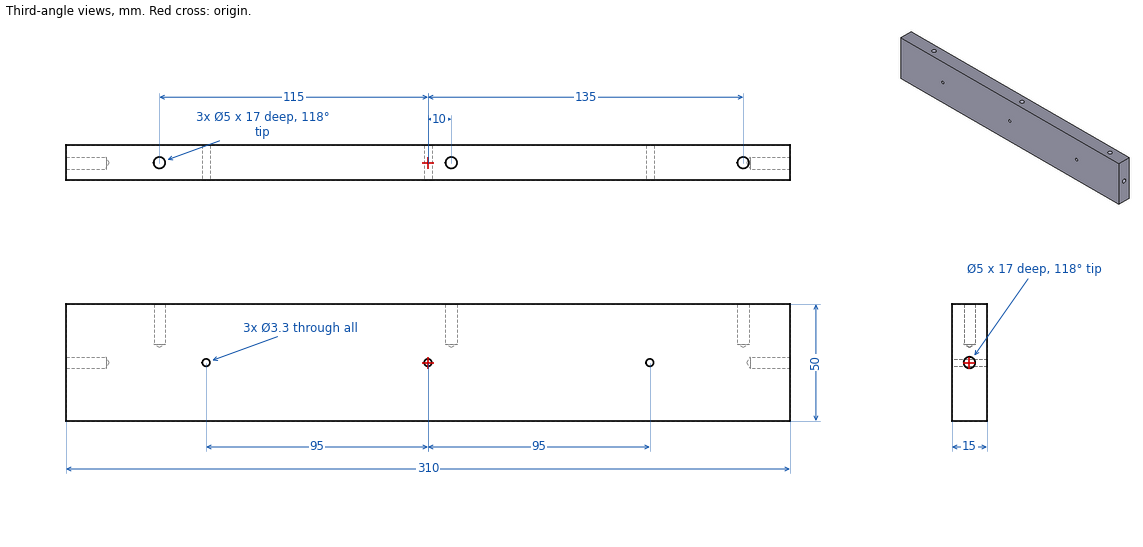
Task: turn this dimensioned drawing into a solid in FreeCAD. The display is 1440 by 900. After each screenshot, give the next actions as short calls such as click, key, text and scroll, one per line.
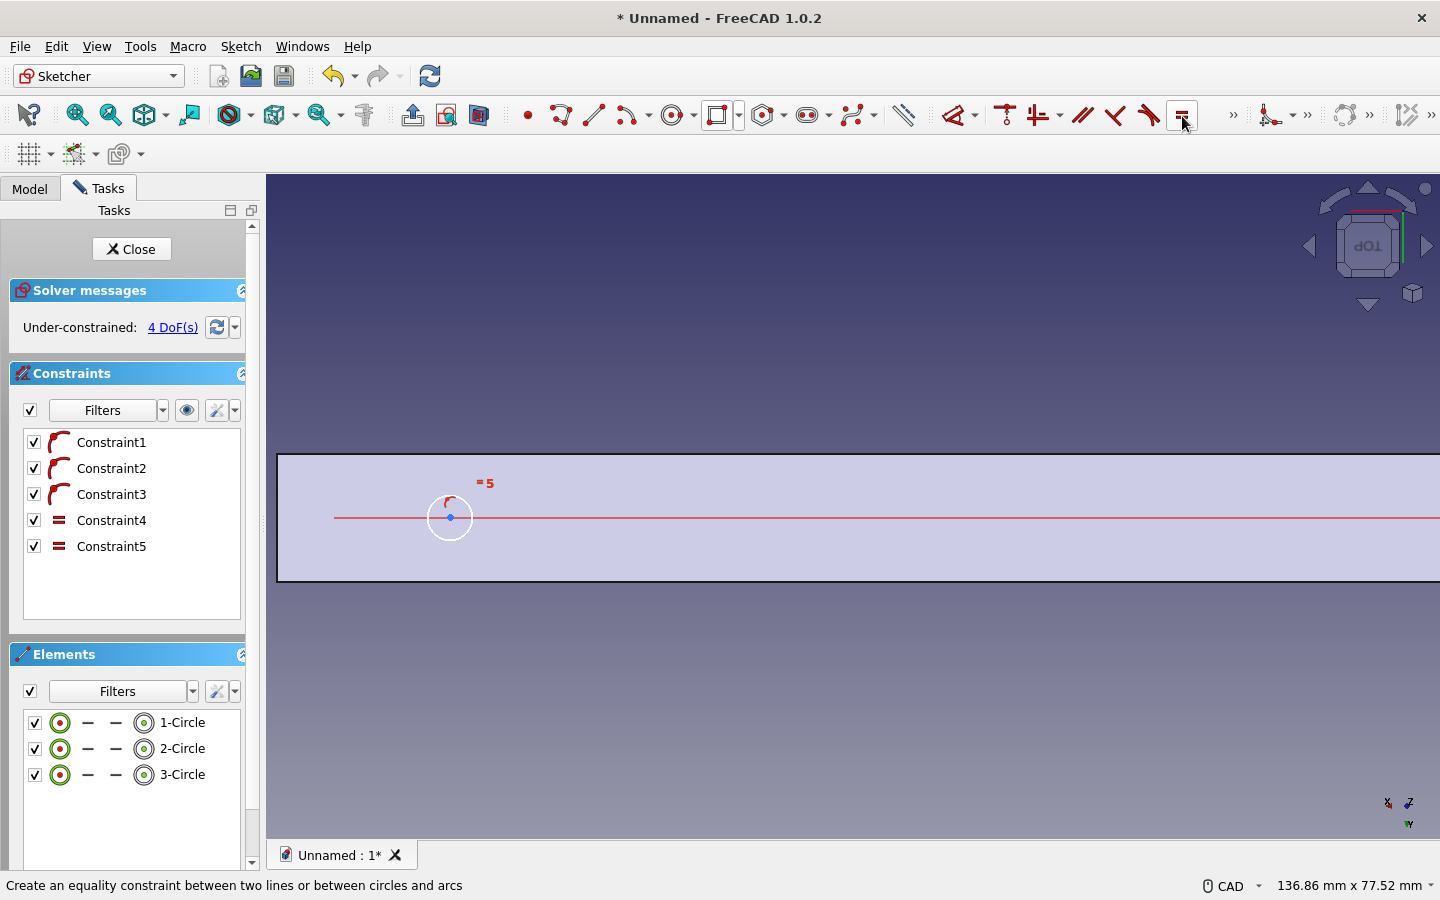
click(952, 116)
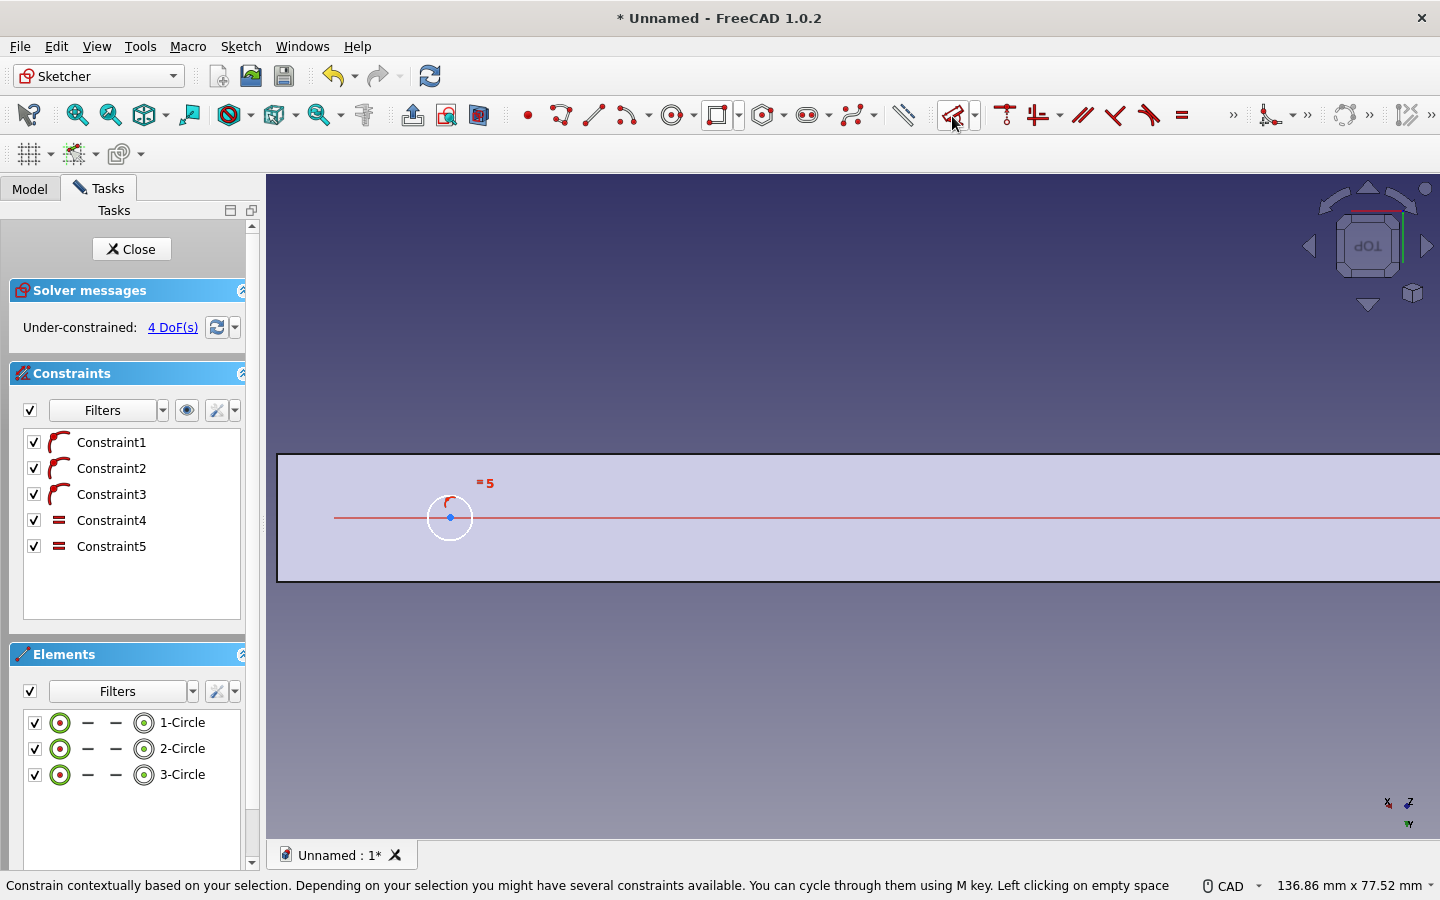
scroll(467, 502, down, 6)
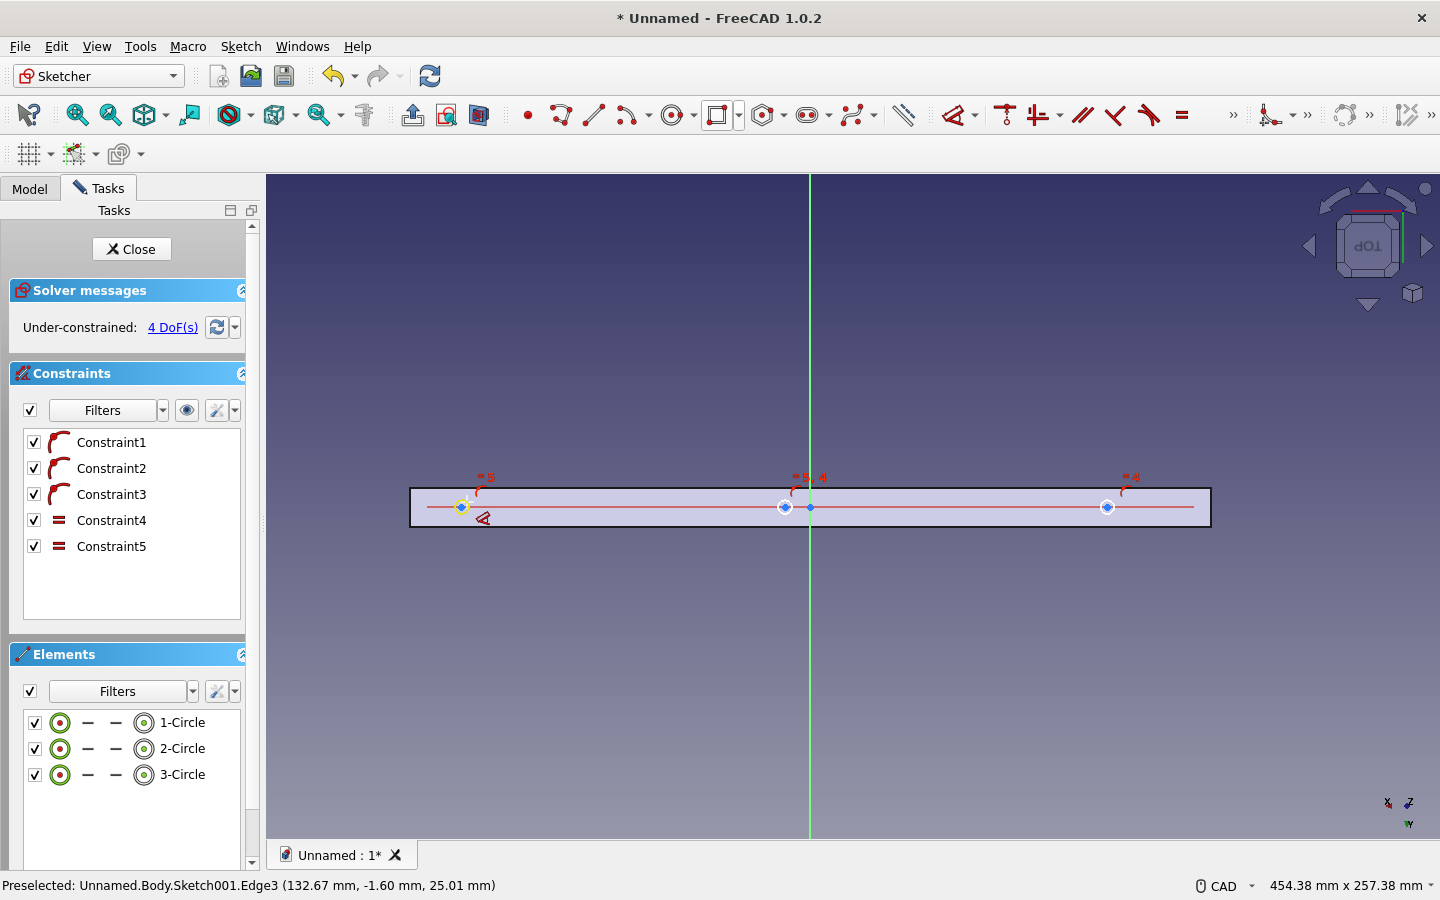
scroll(1112, 502, up, 6)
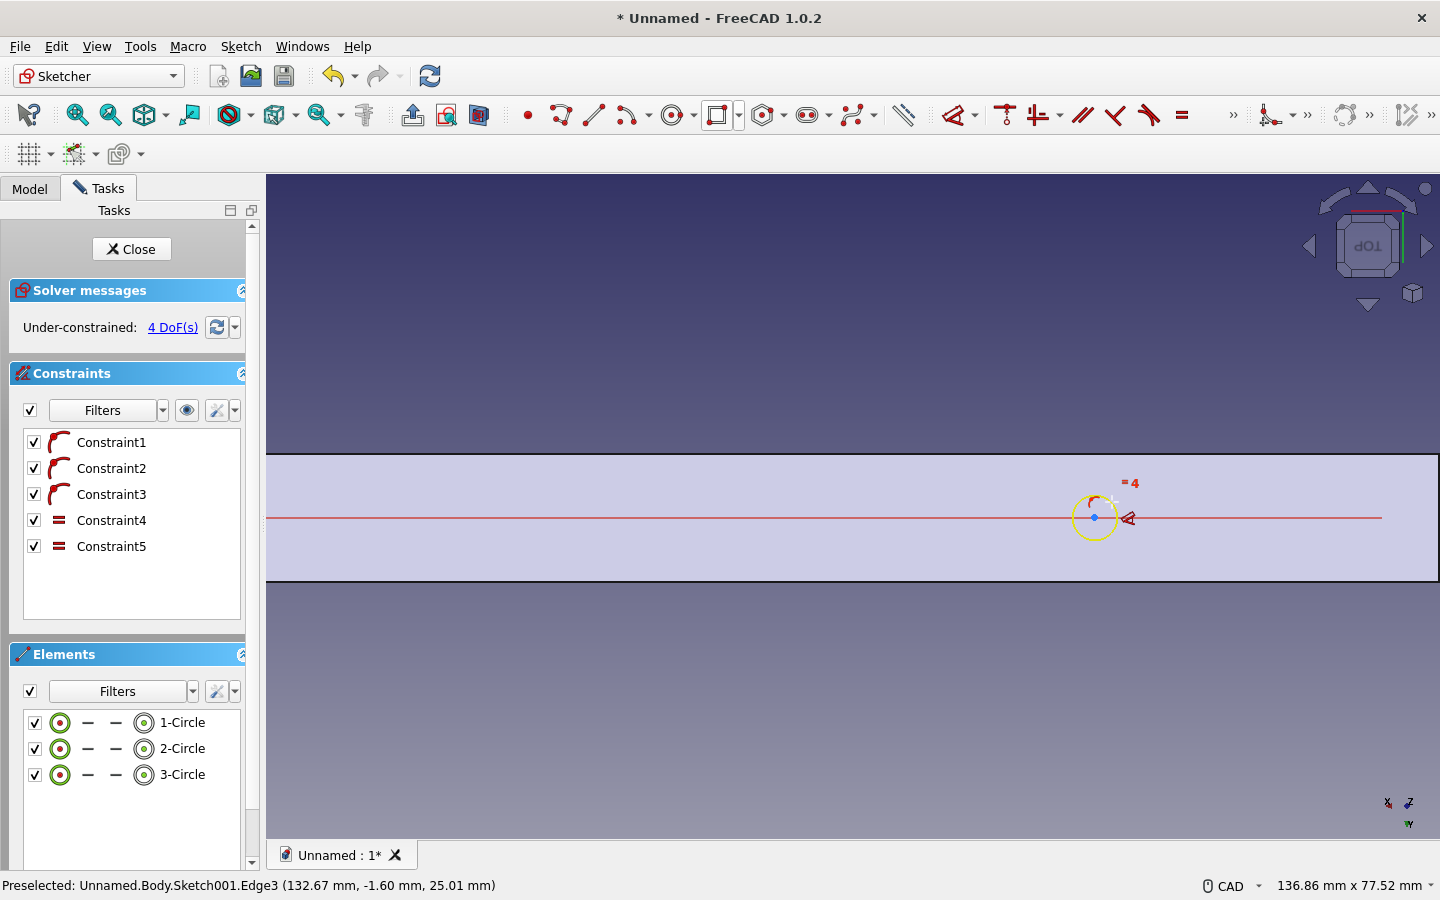
click(1111, 502)
click(1134, 479)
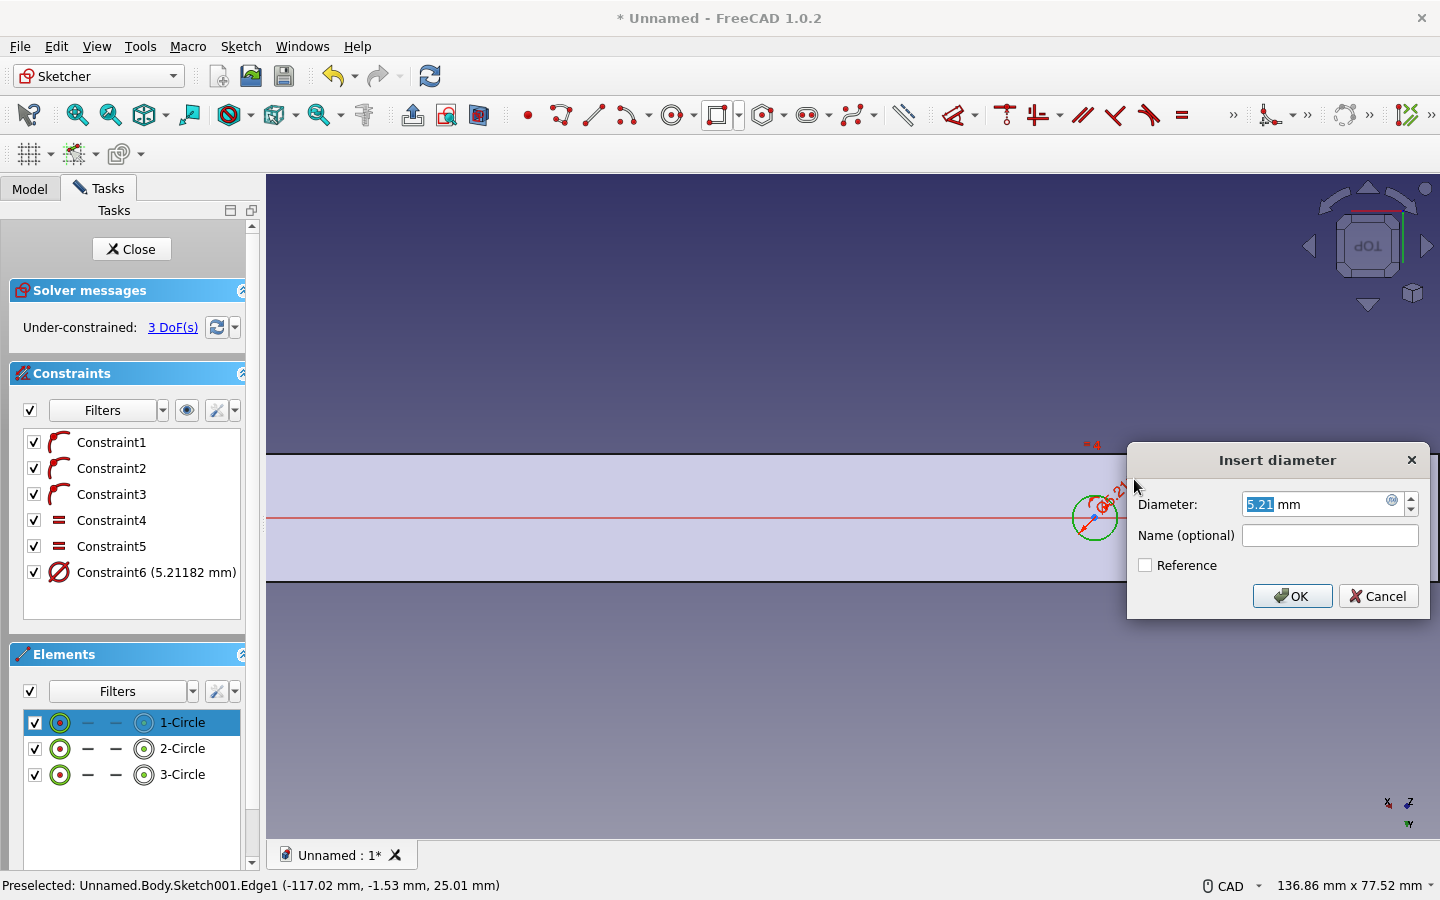
text(5)
key(Return)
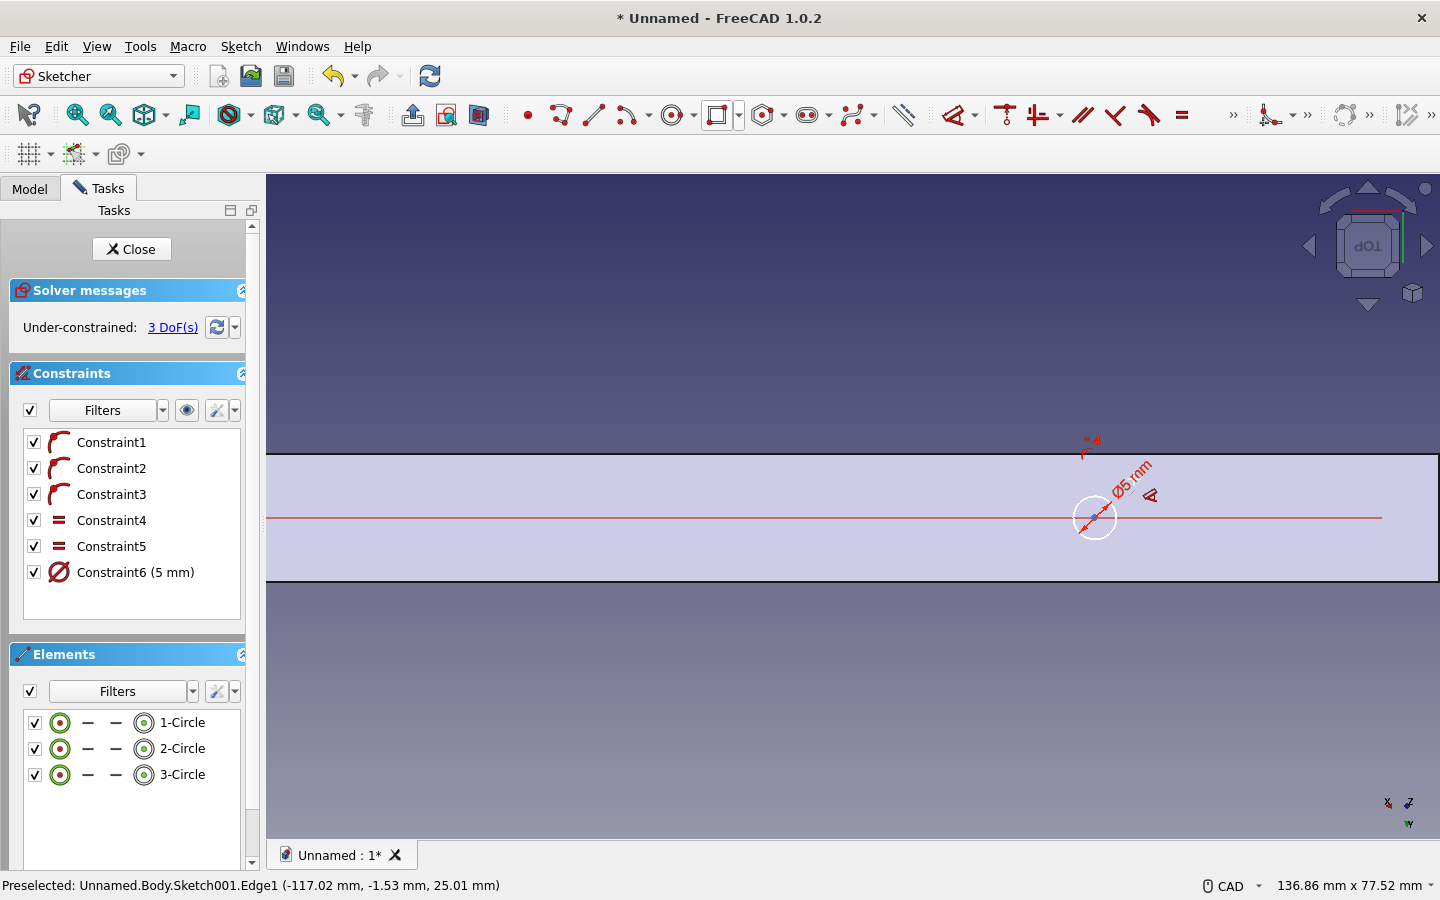
scroll(1113, 502, down, 6)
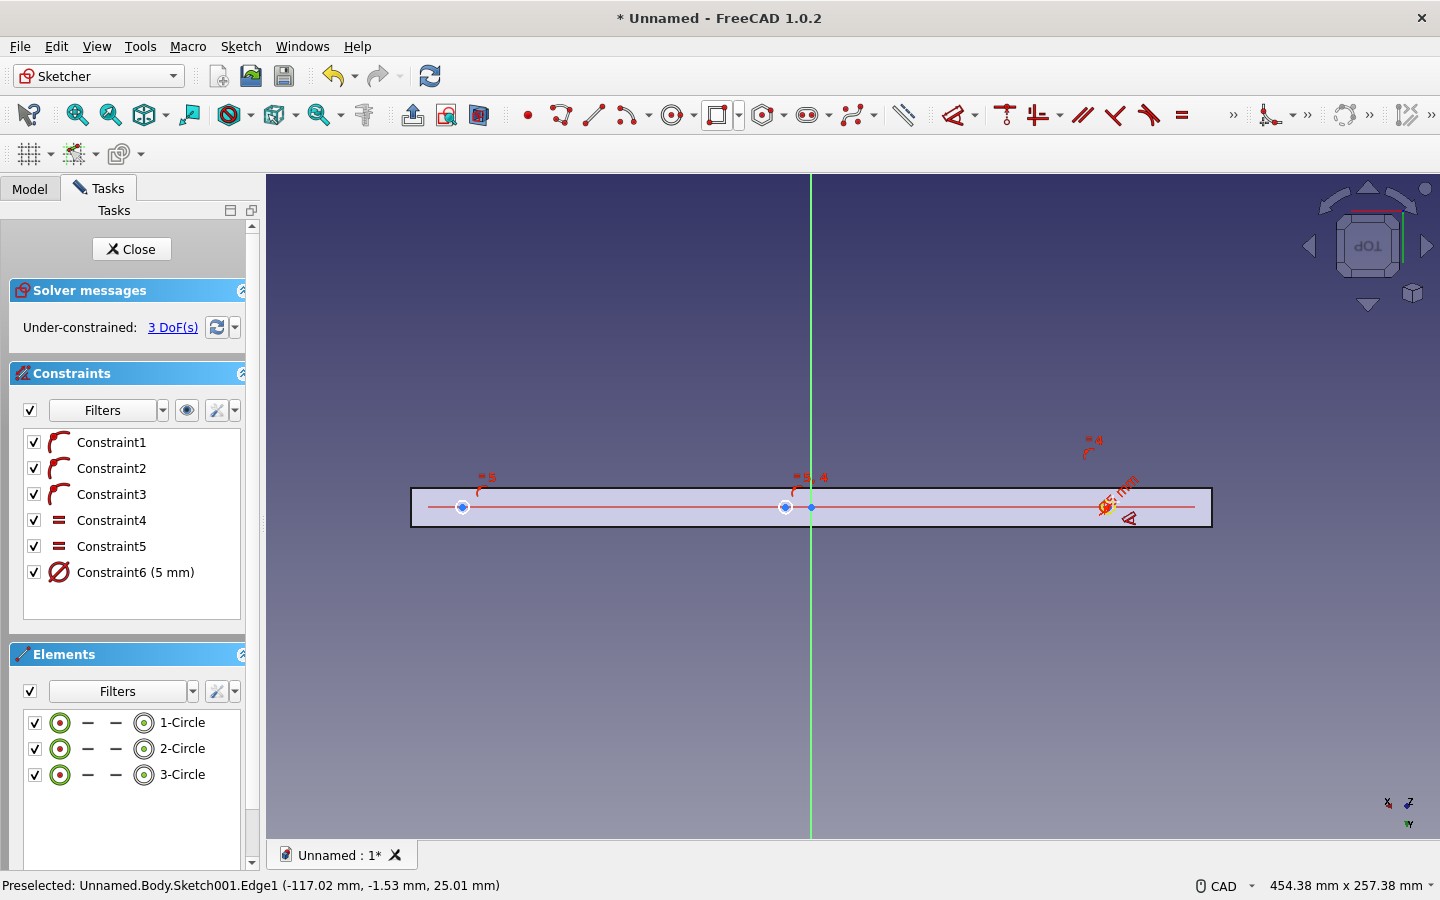
scroll(786, 507, up, 3)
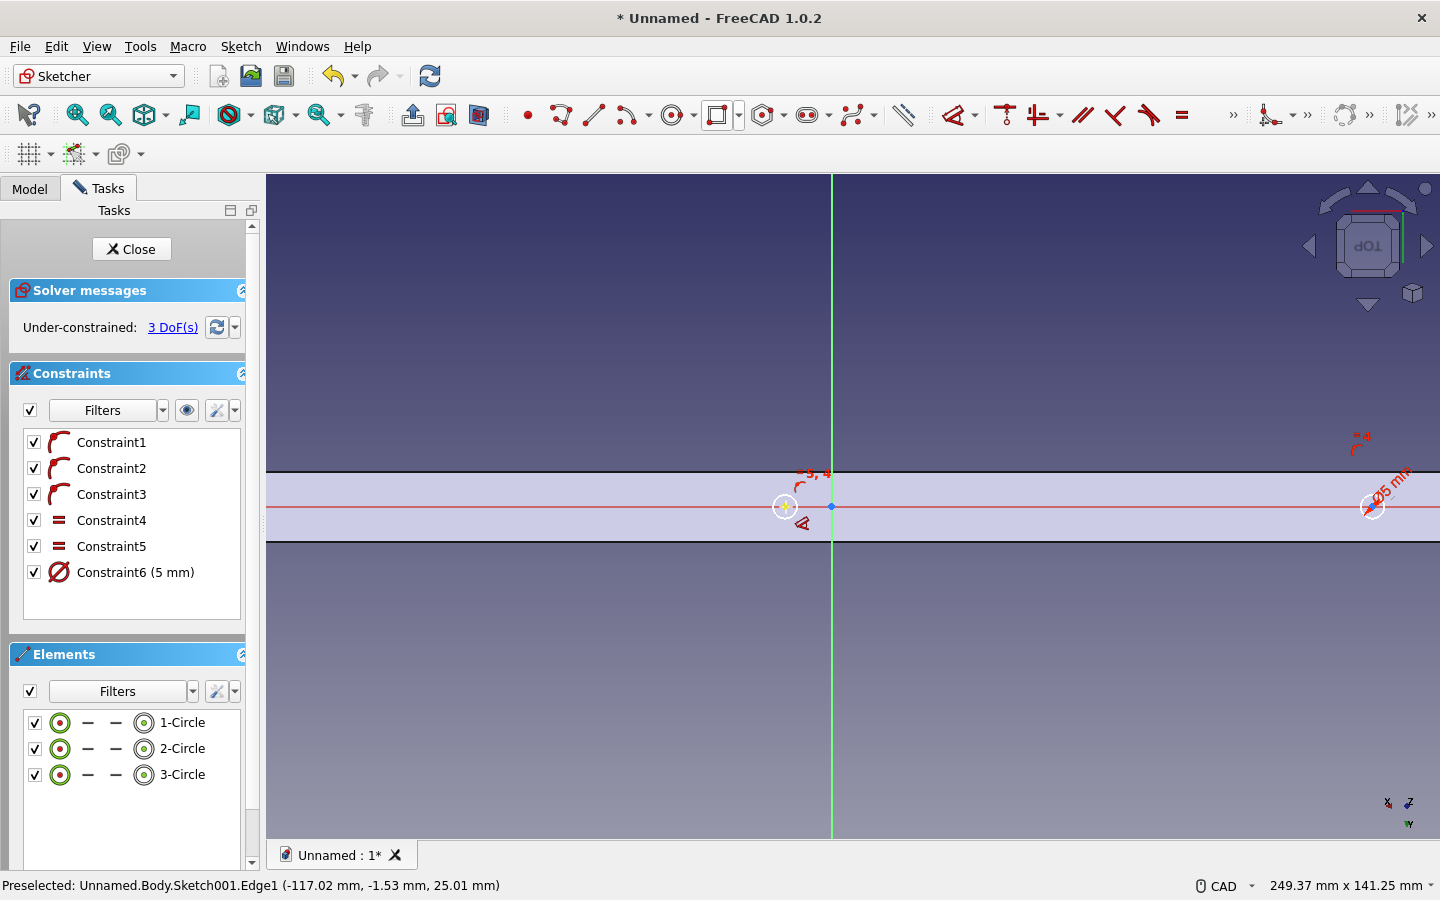
click(785, 507)
click(808, 541)